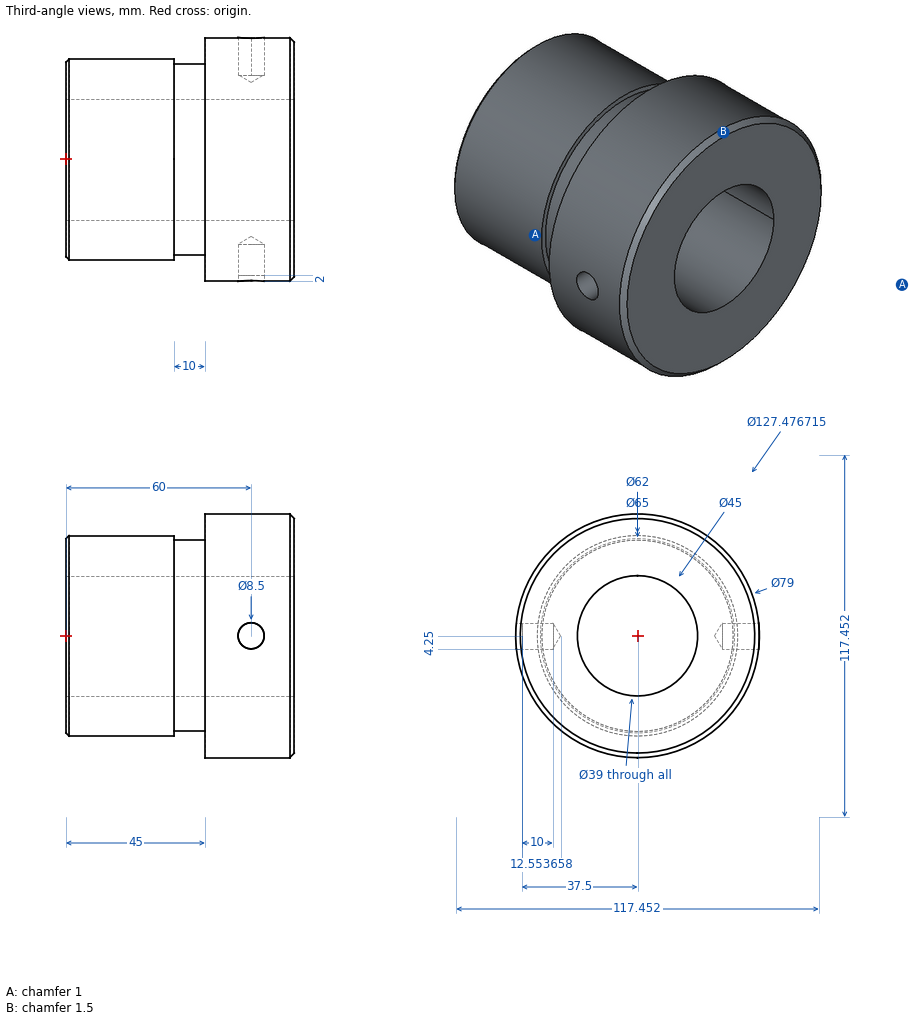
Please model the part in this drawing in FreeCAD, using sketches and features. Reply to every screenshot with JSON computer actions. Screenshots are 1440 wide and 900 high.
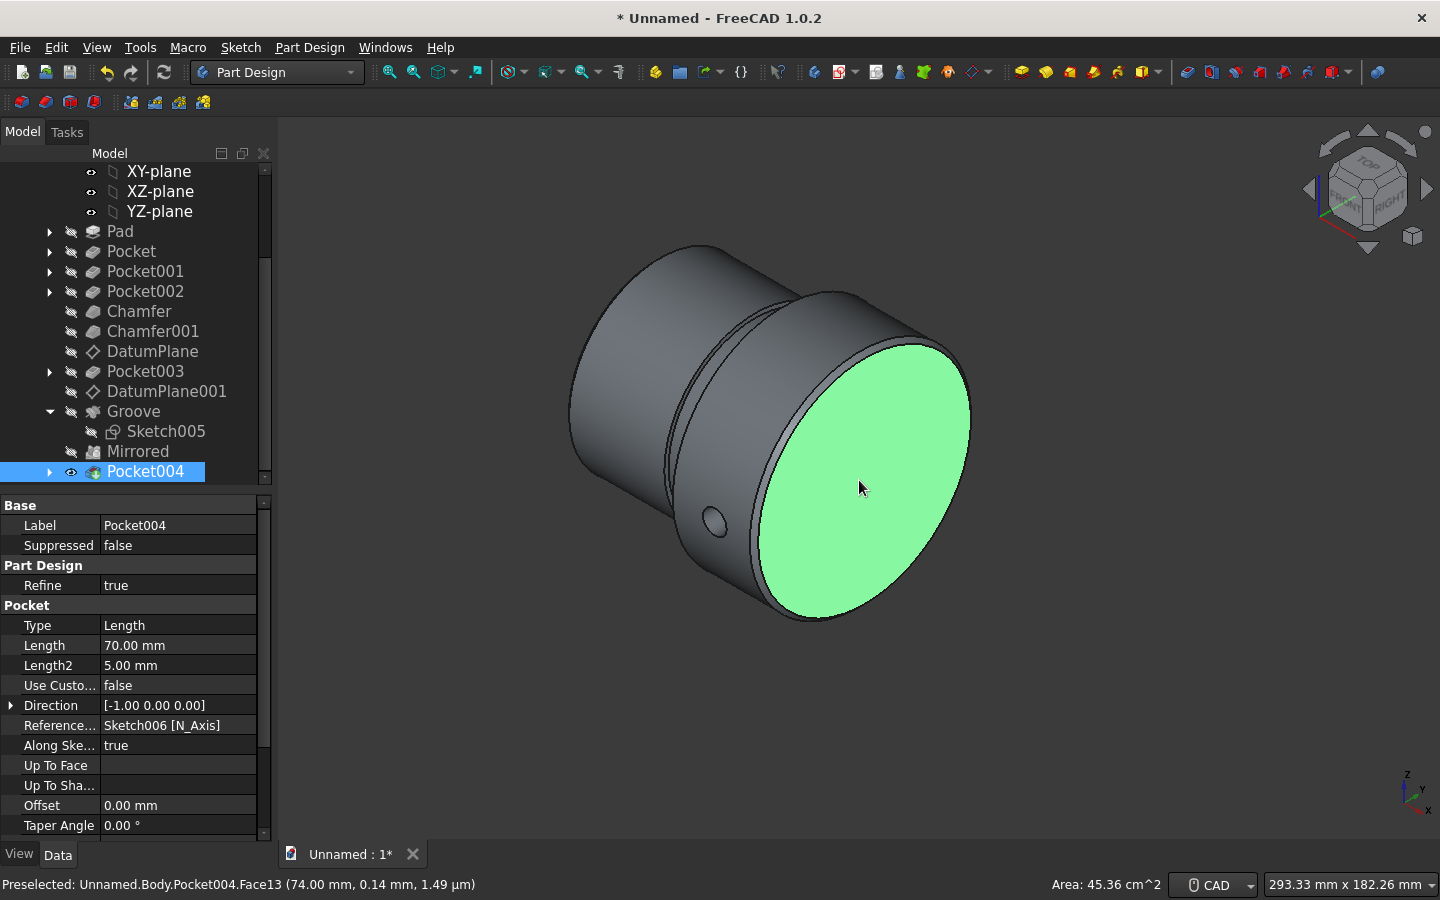
{"action": "left_click", "coordinate": [840, 72]}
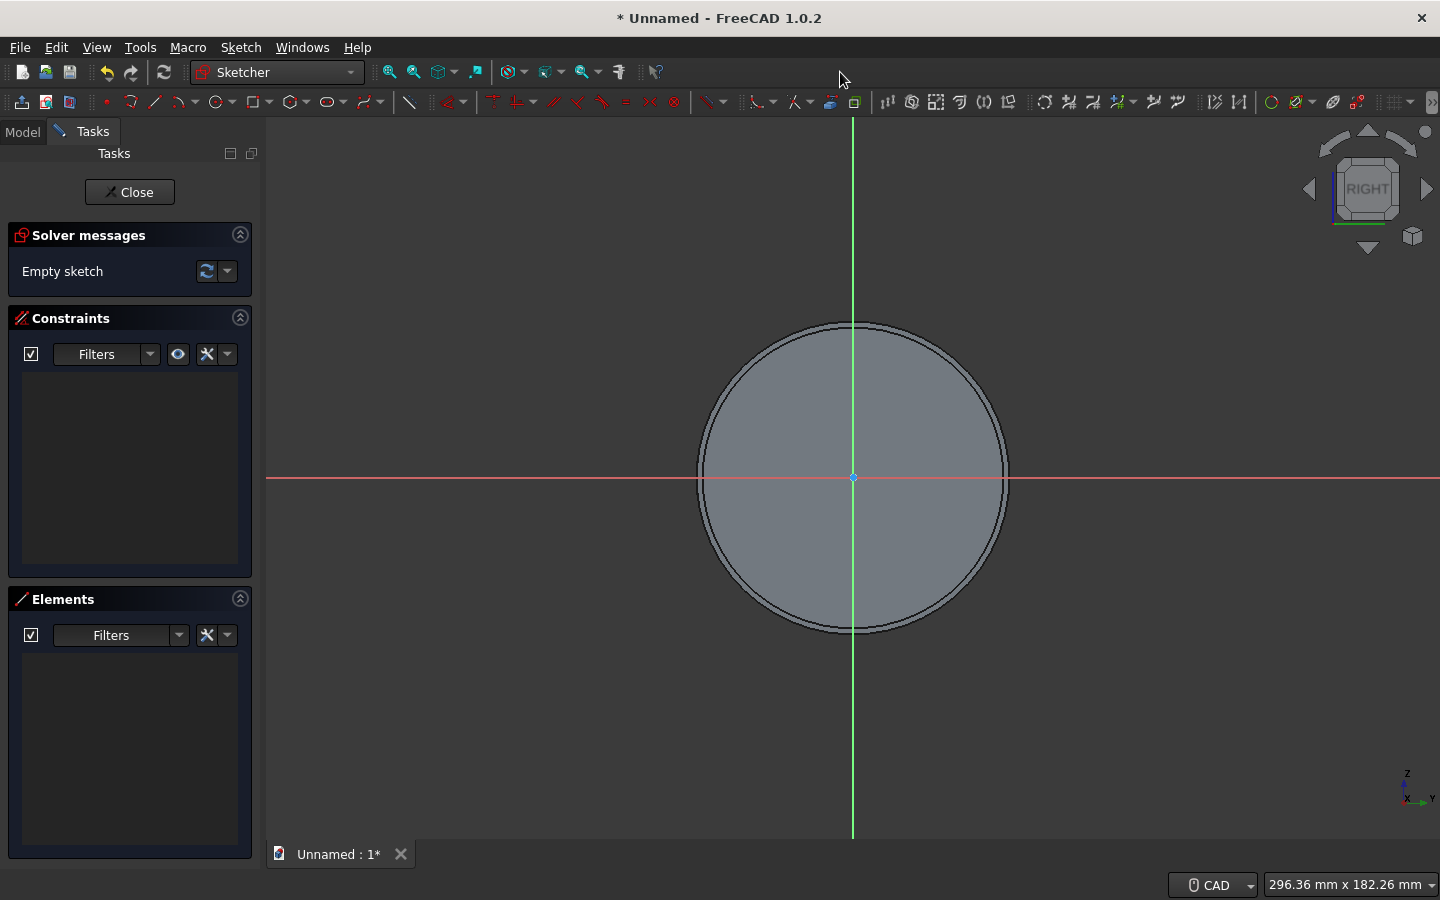
{"action": "scroll", "coordinate": [883, 478], "scroll_direction": "up", "scroll_amount": 6}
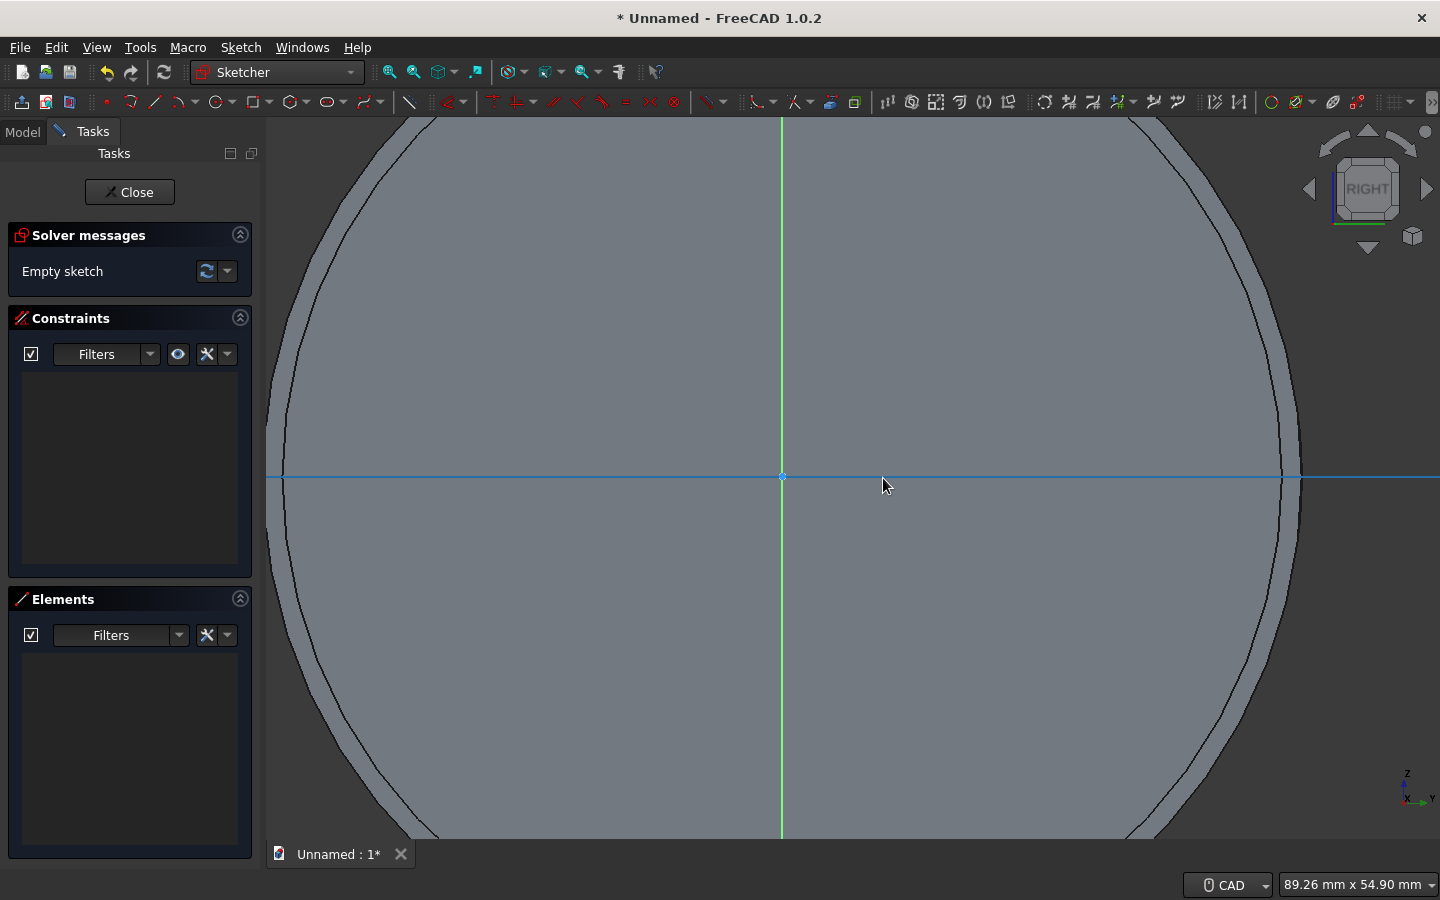
{"action": "key", "text": "g c"}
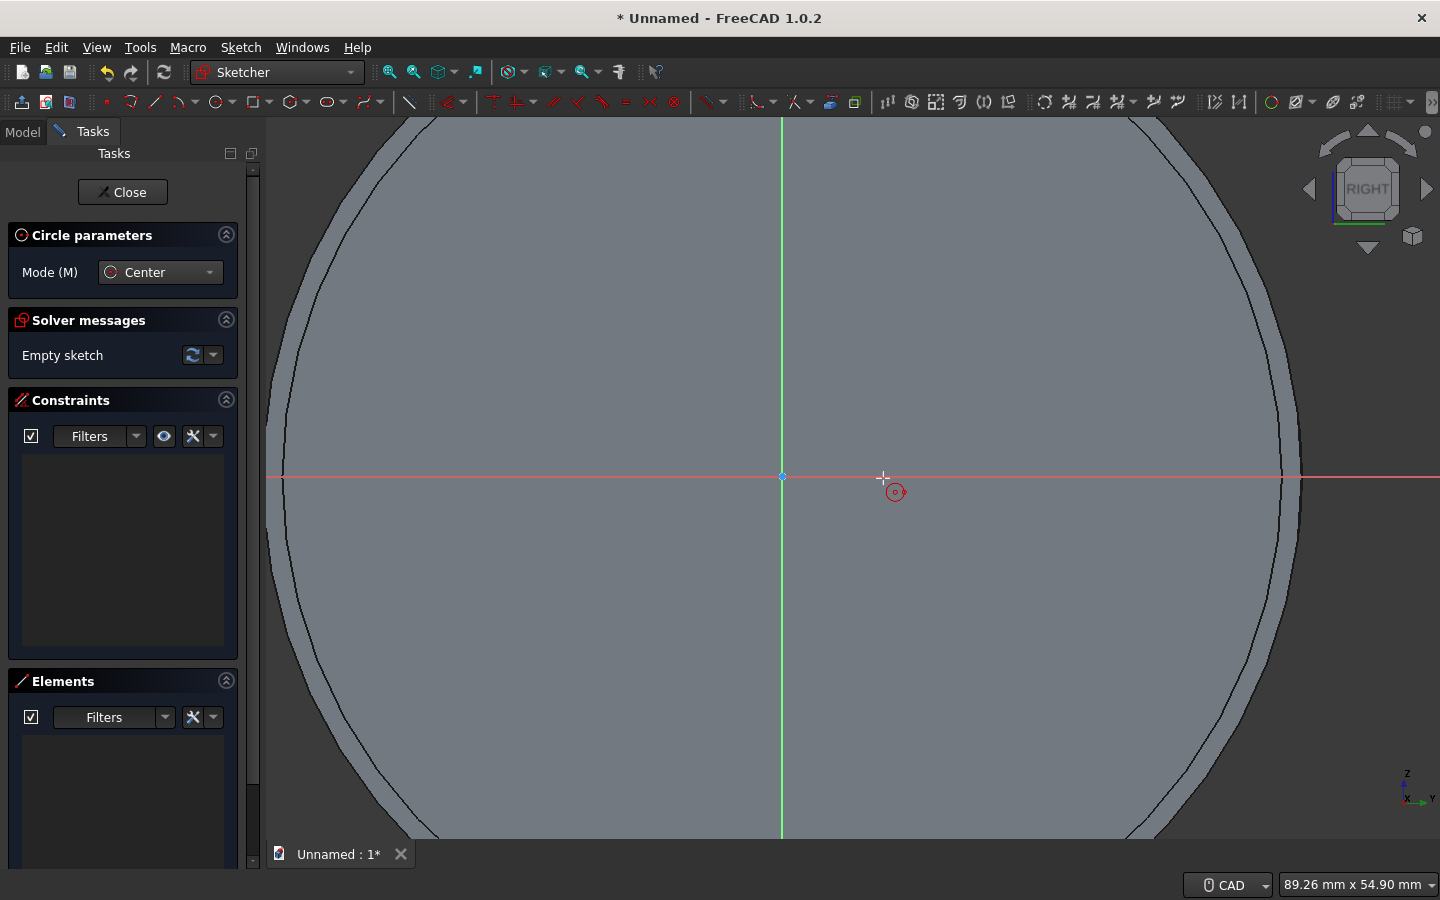
{"action": "left_click", "coordinate": [782, 477]}
{"action": "mouse_move", "coordinate": [964, 295]}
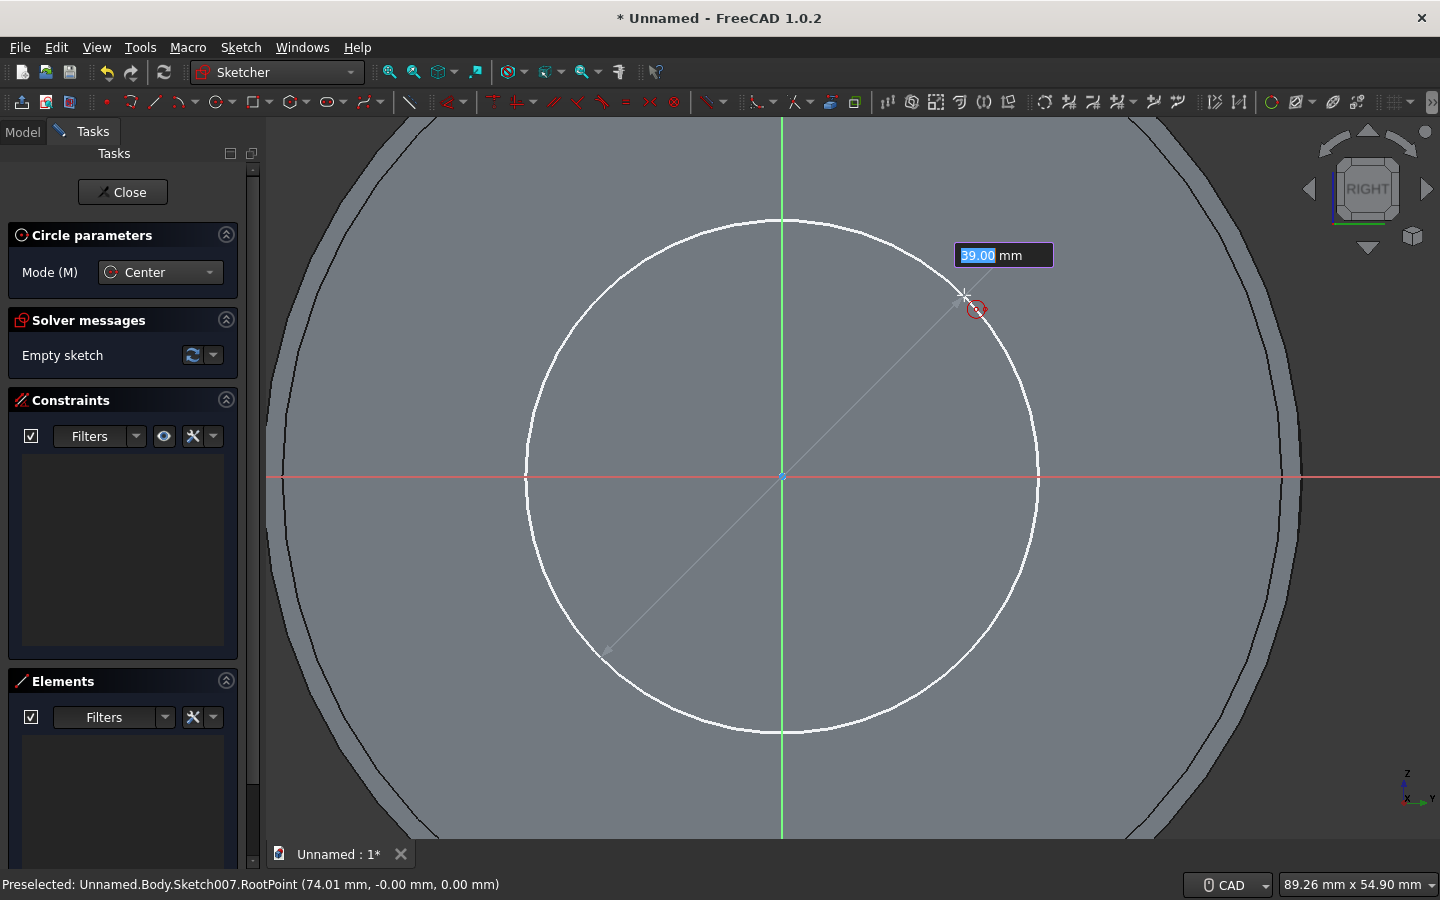
{"action": "type", "text": "39"}
{"action": "key", "text": "Return"}
{"action": "key", "text": "Escape"}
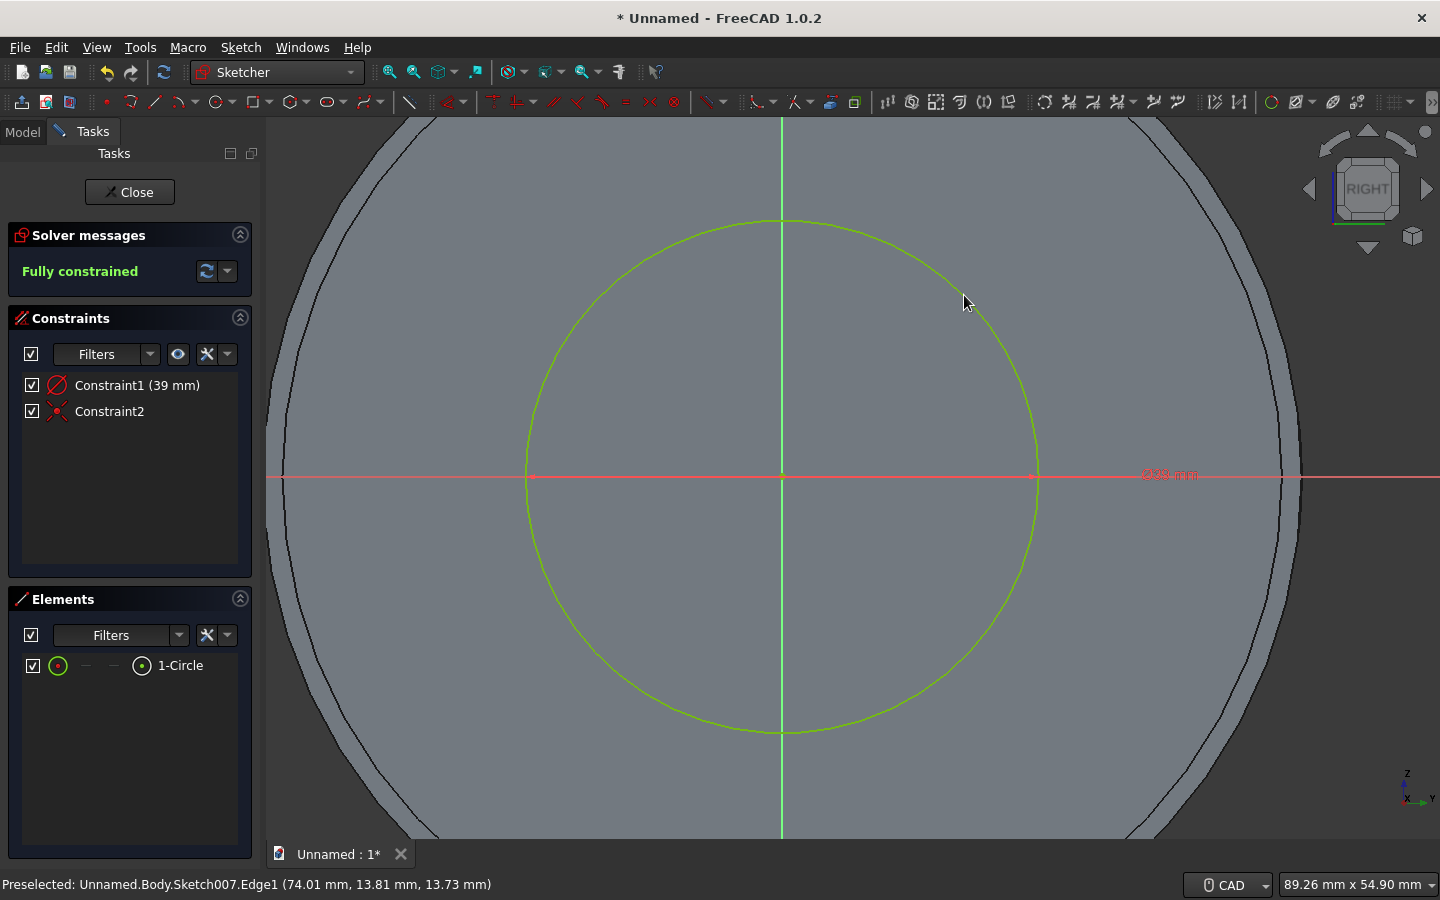
{"action": "left_click", "coordinate": [130, 192]}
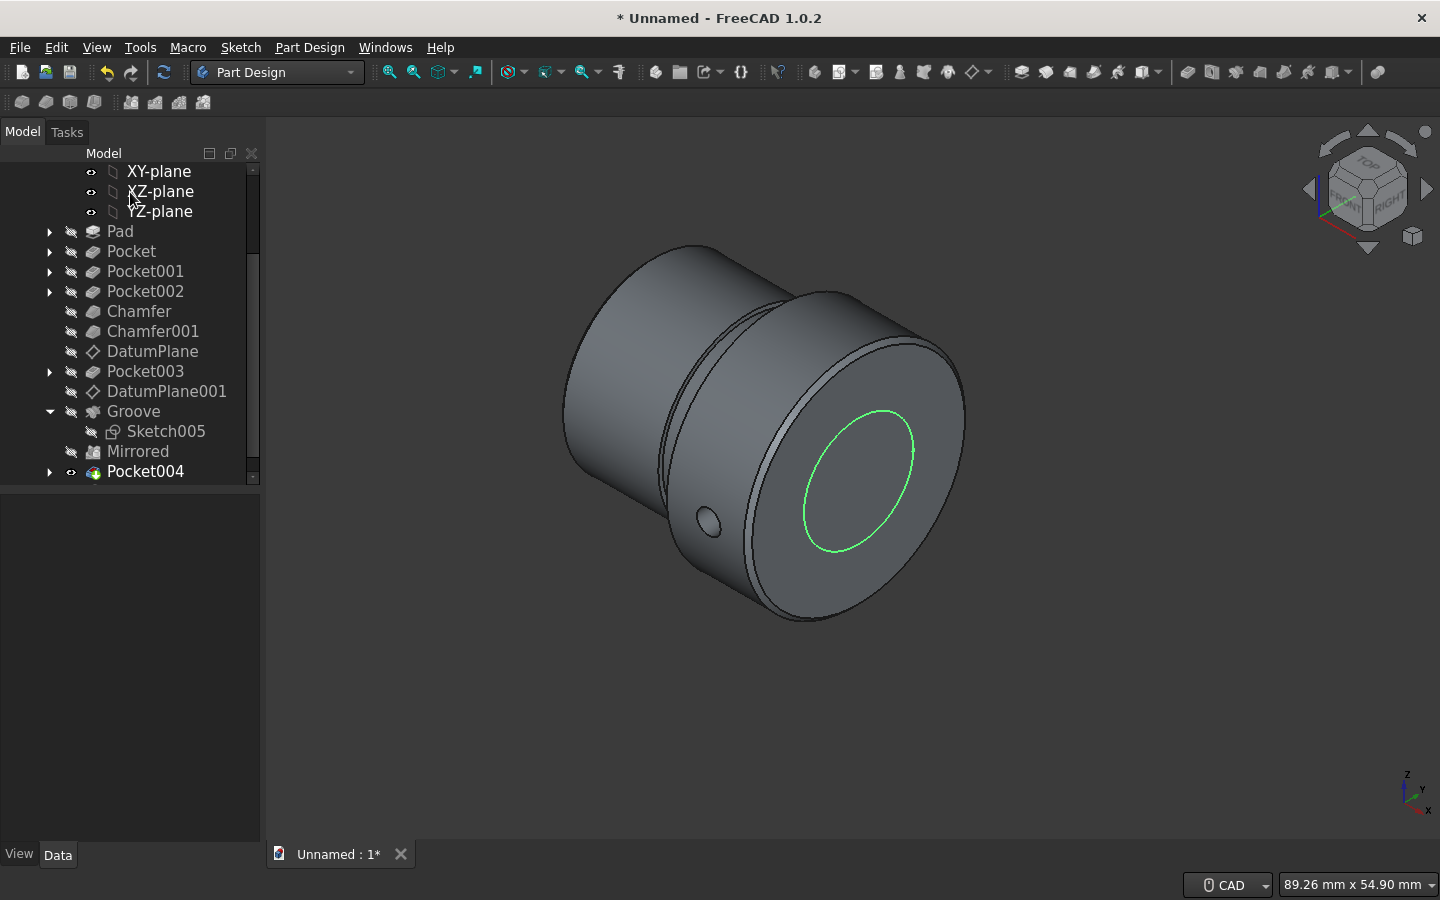
{"action": "left_click", "coordinate": [1212, 72]}